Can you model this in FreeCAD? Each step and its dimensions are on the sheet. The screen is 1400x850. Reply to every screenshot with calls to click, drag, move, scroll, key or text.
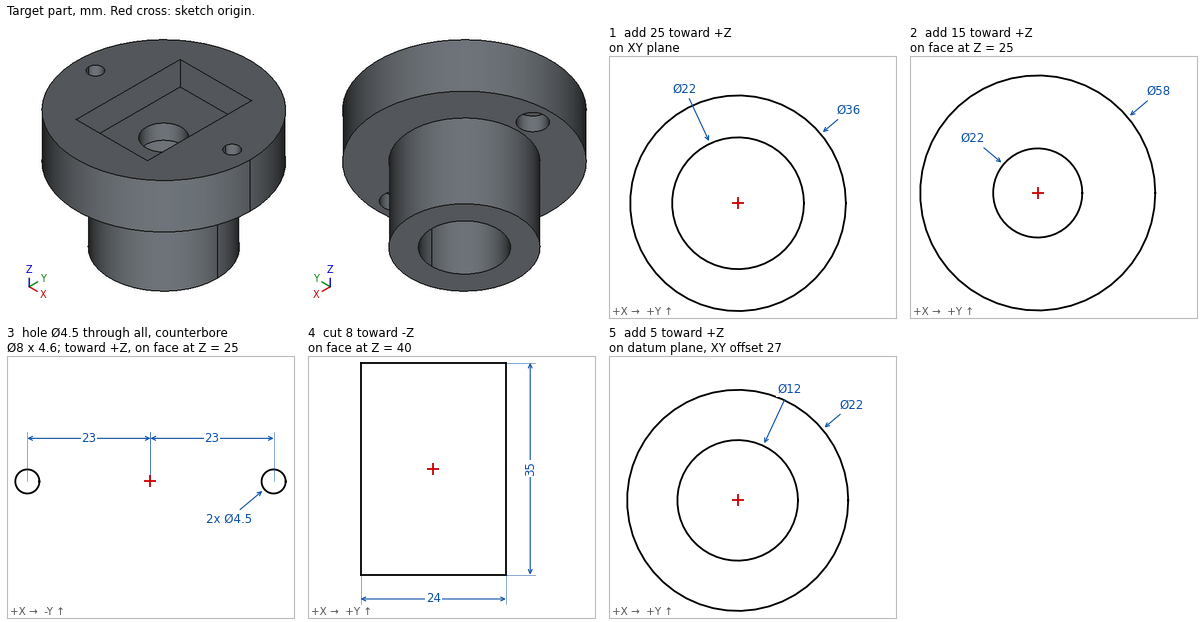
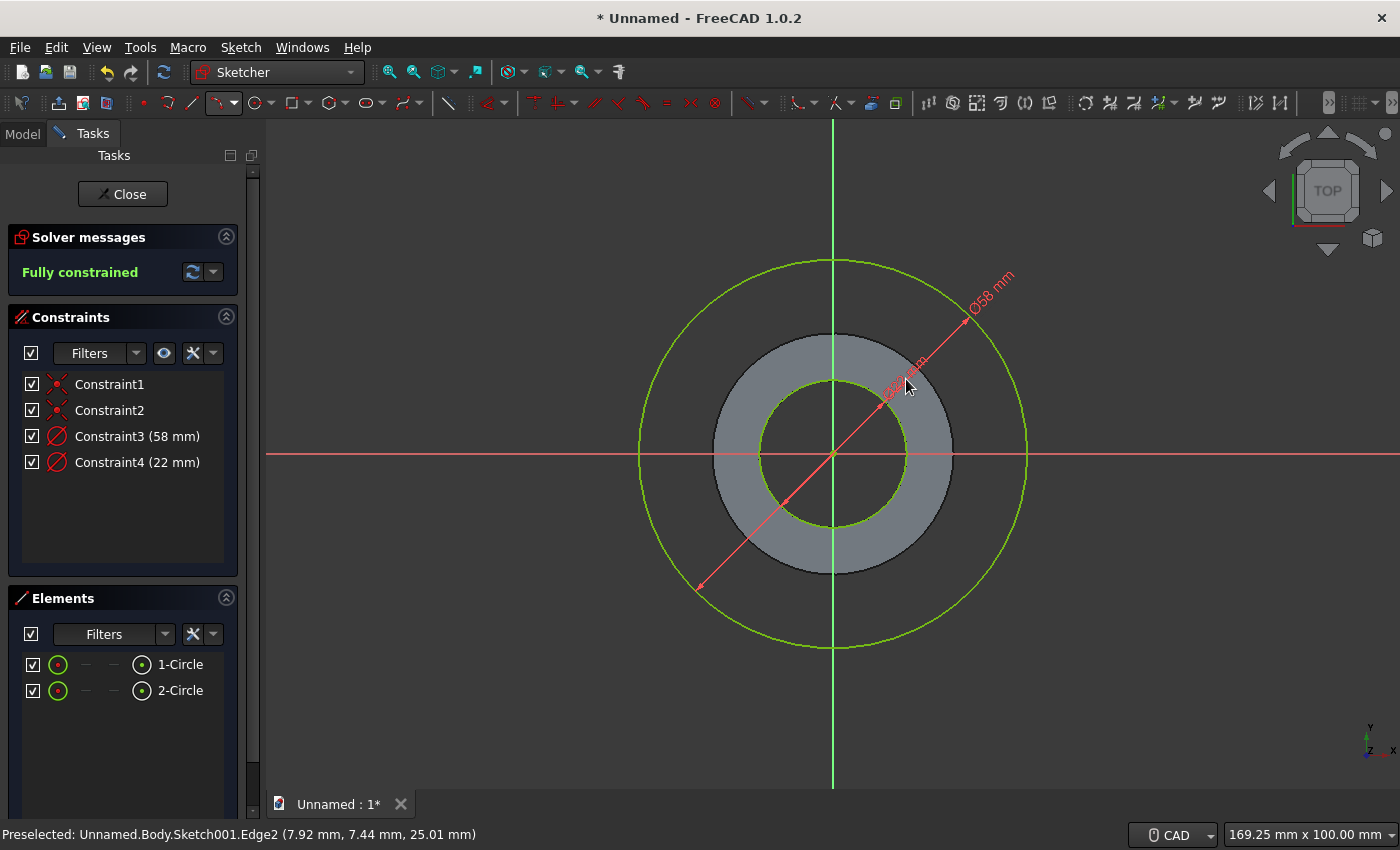
click(123, 194)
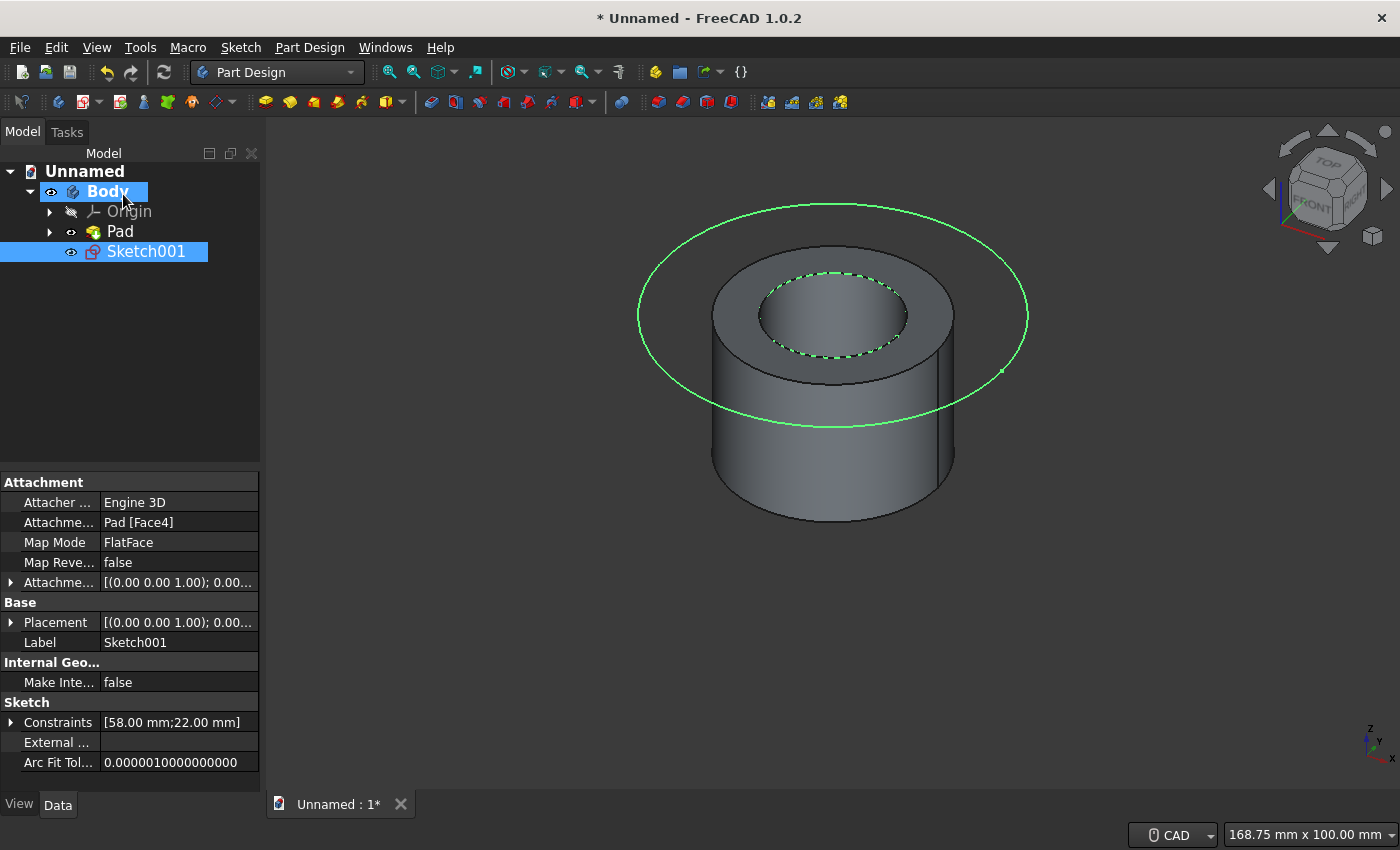
click(266, 102)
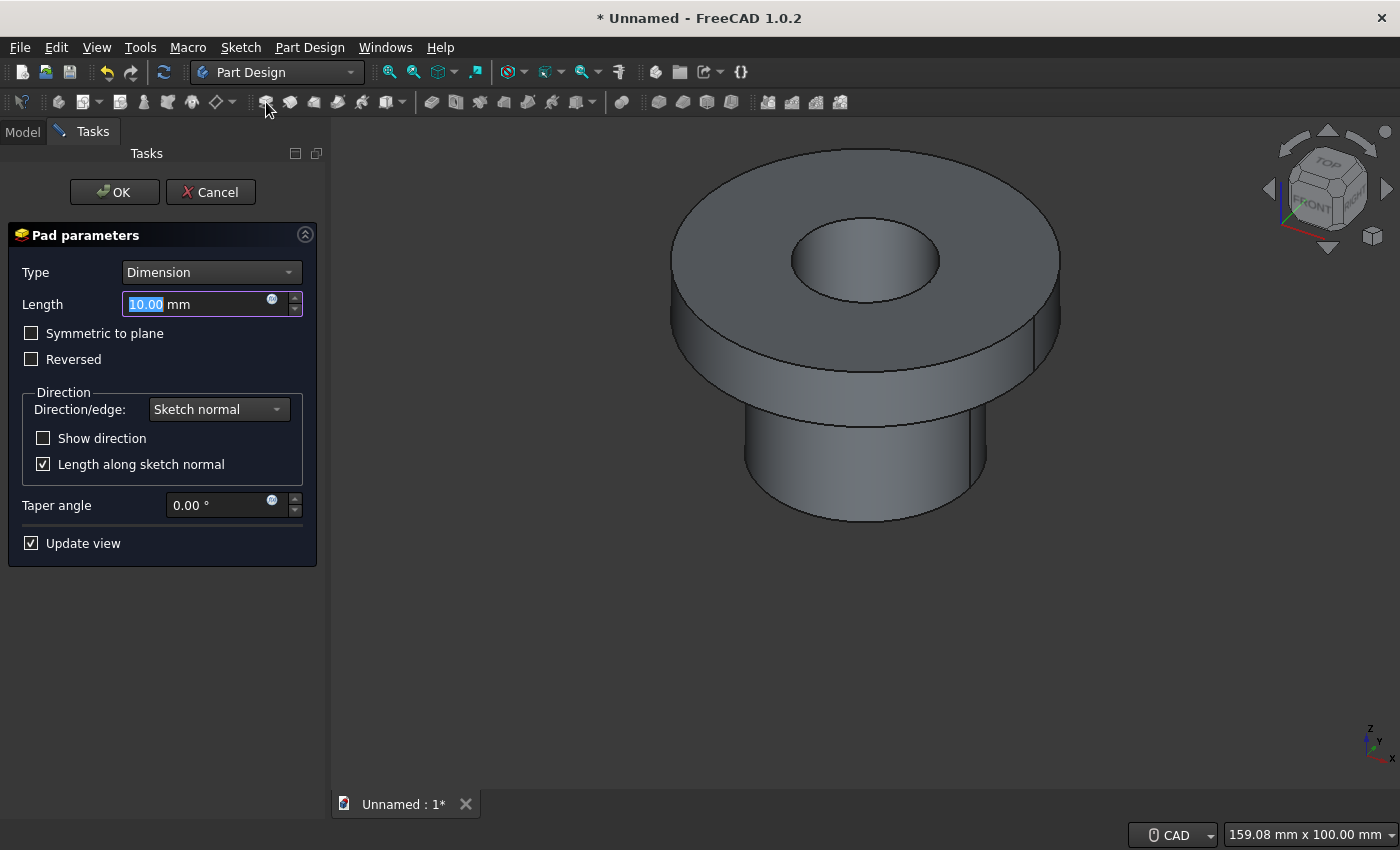
text(15)
key(Tab)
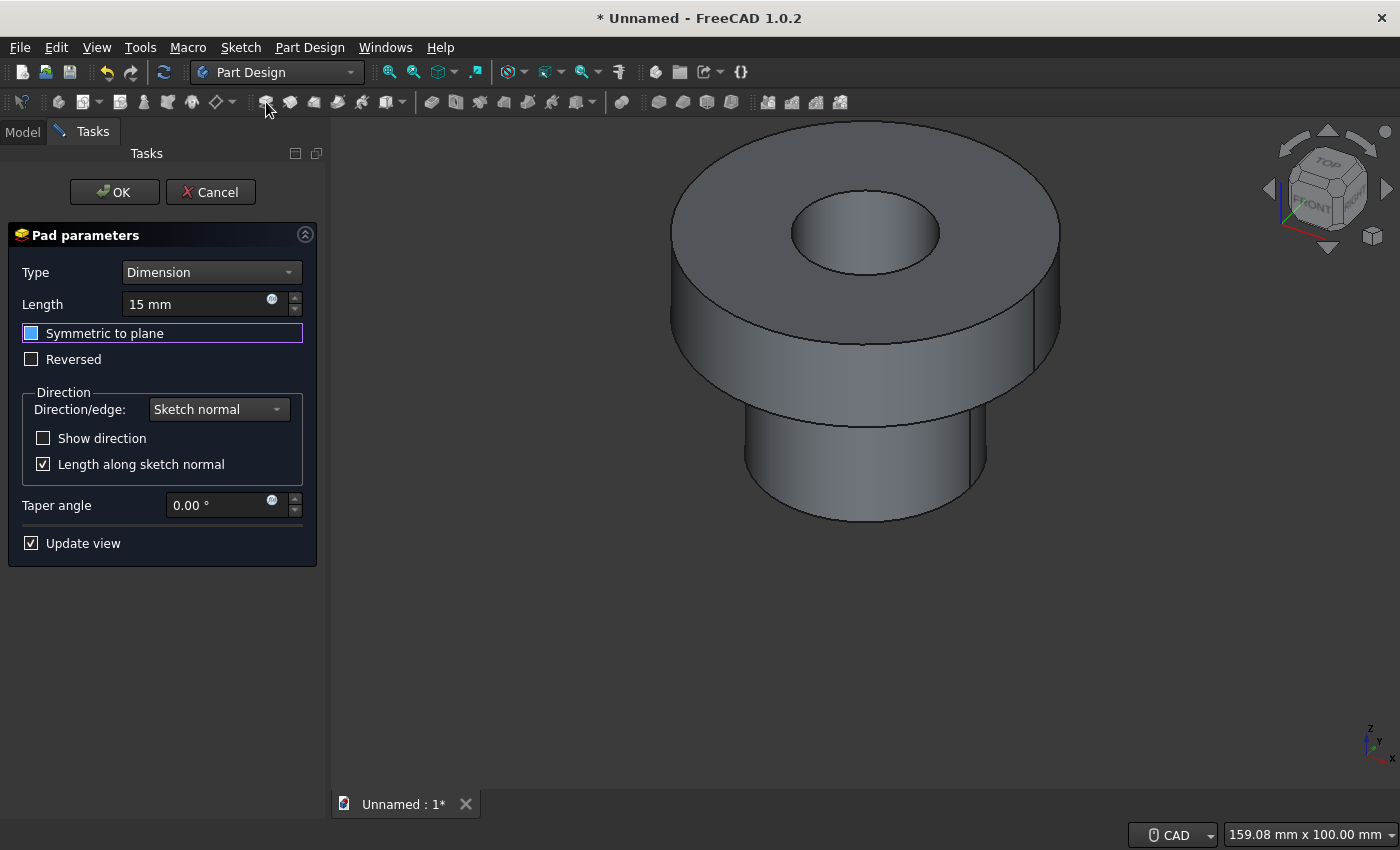
click(115, 192)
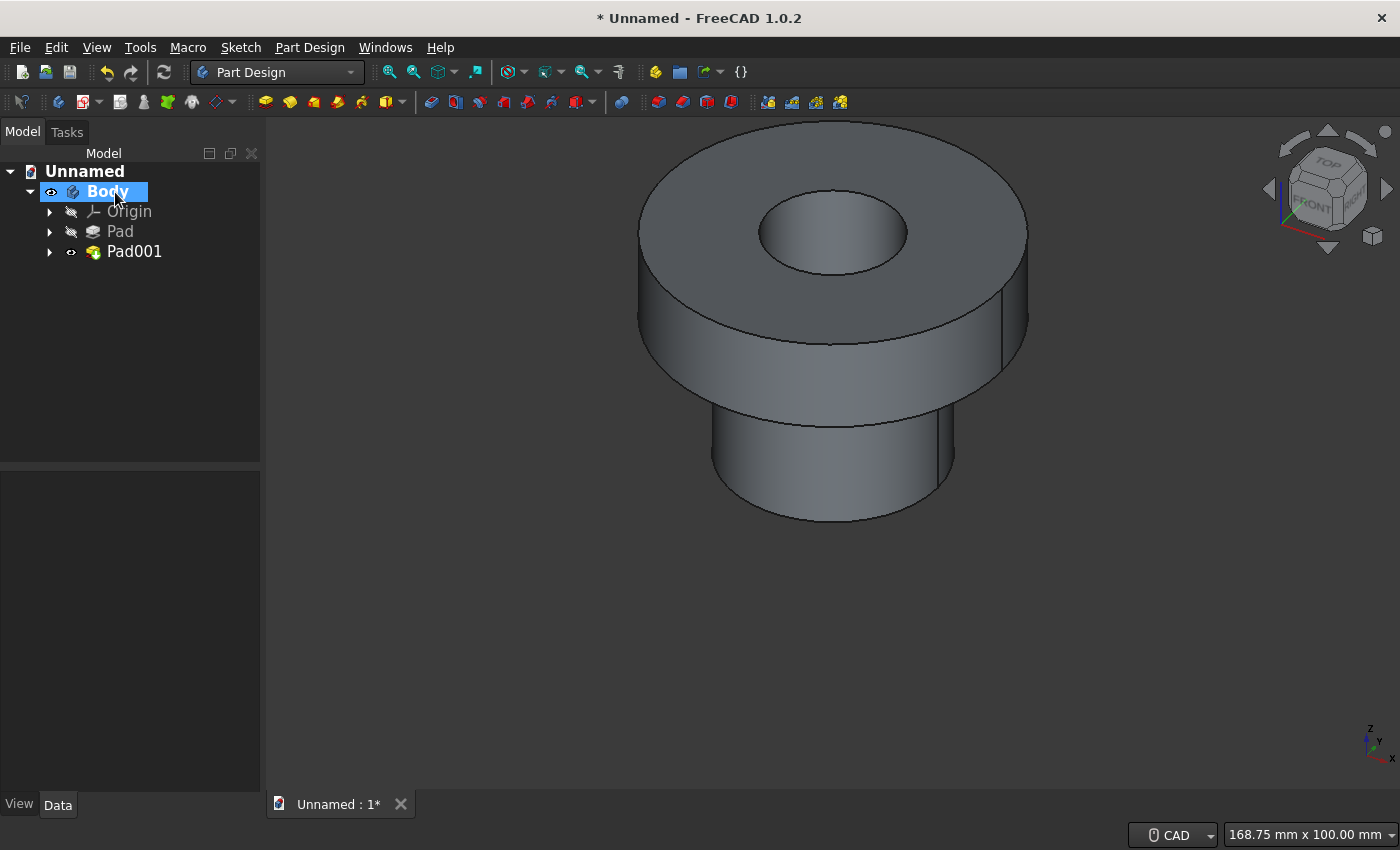
key(v)
key(f)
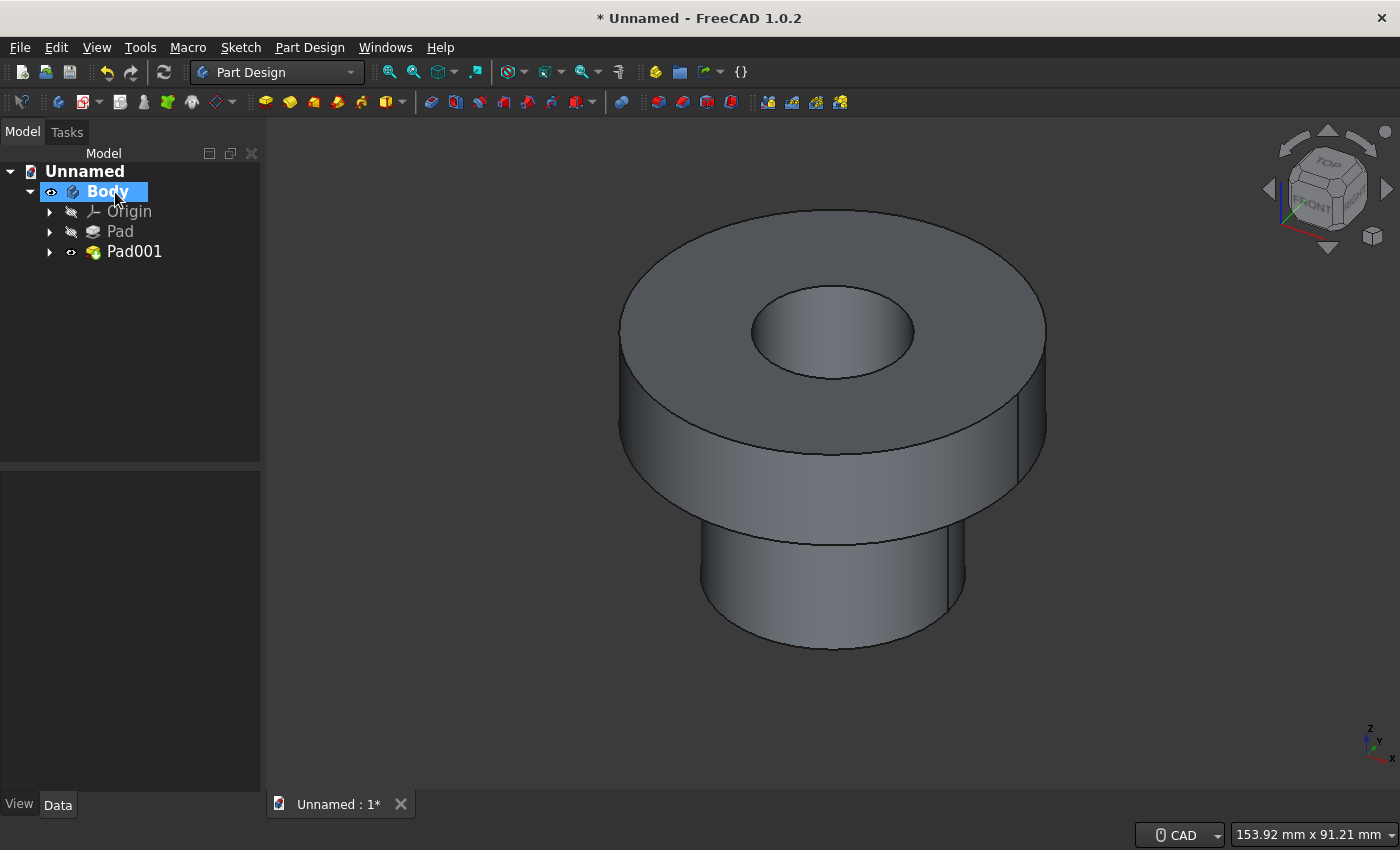
key(5)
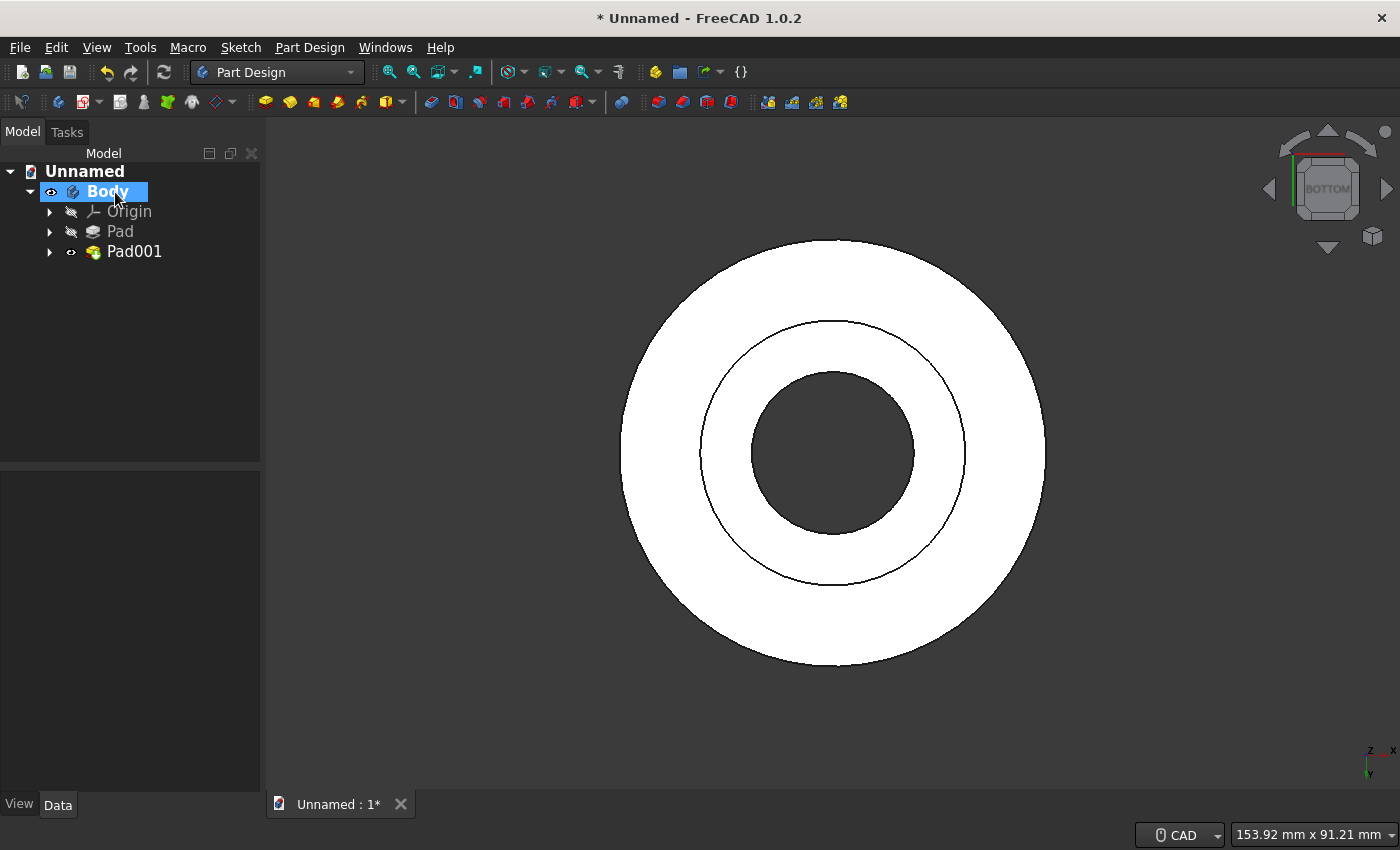
click(955, 330)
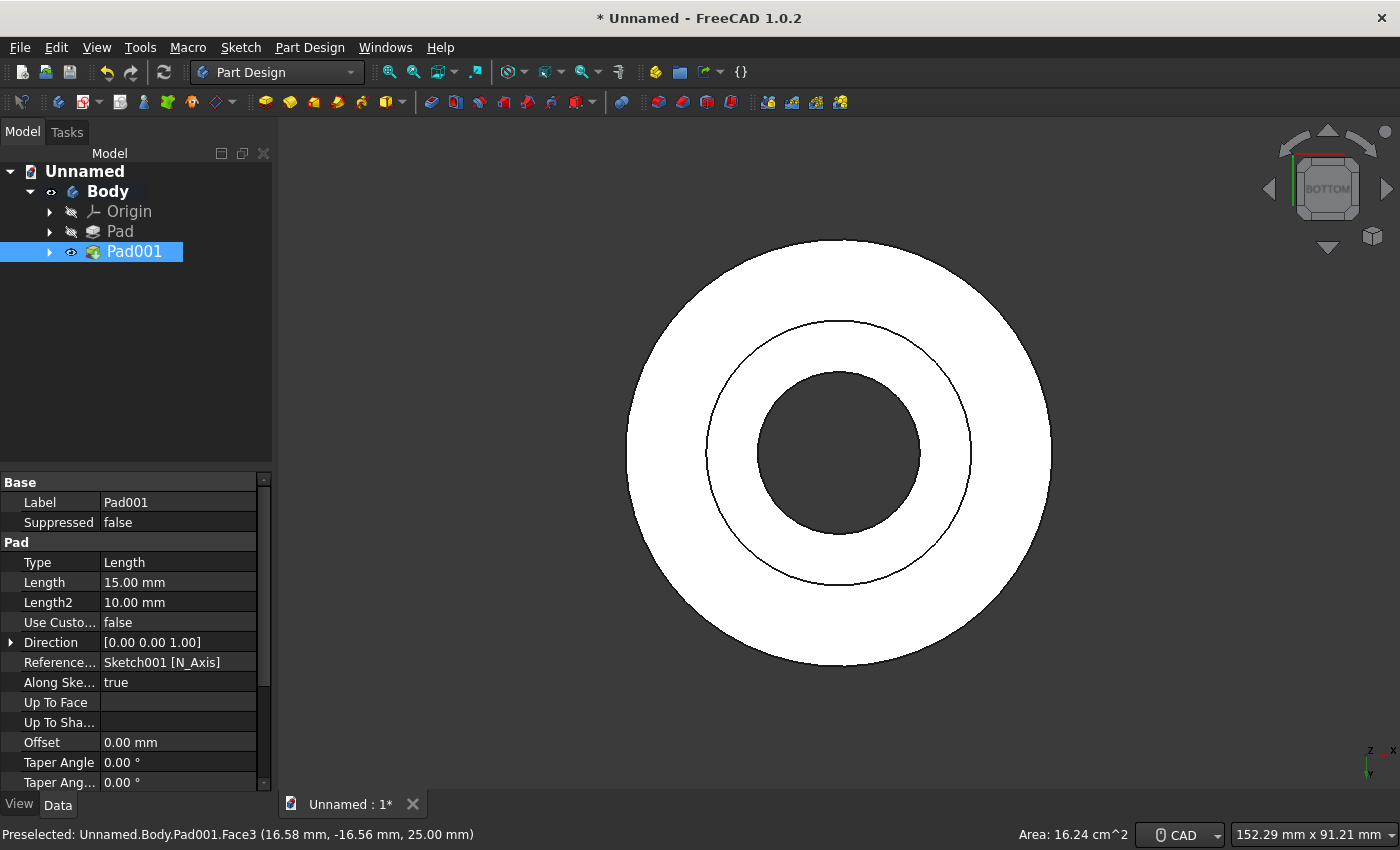
click(84, 102)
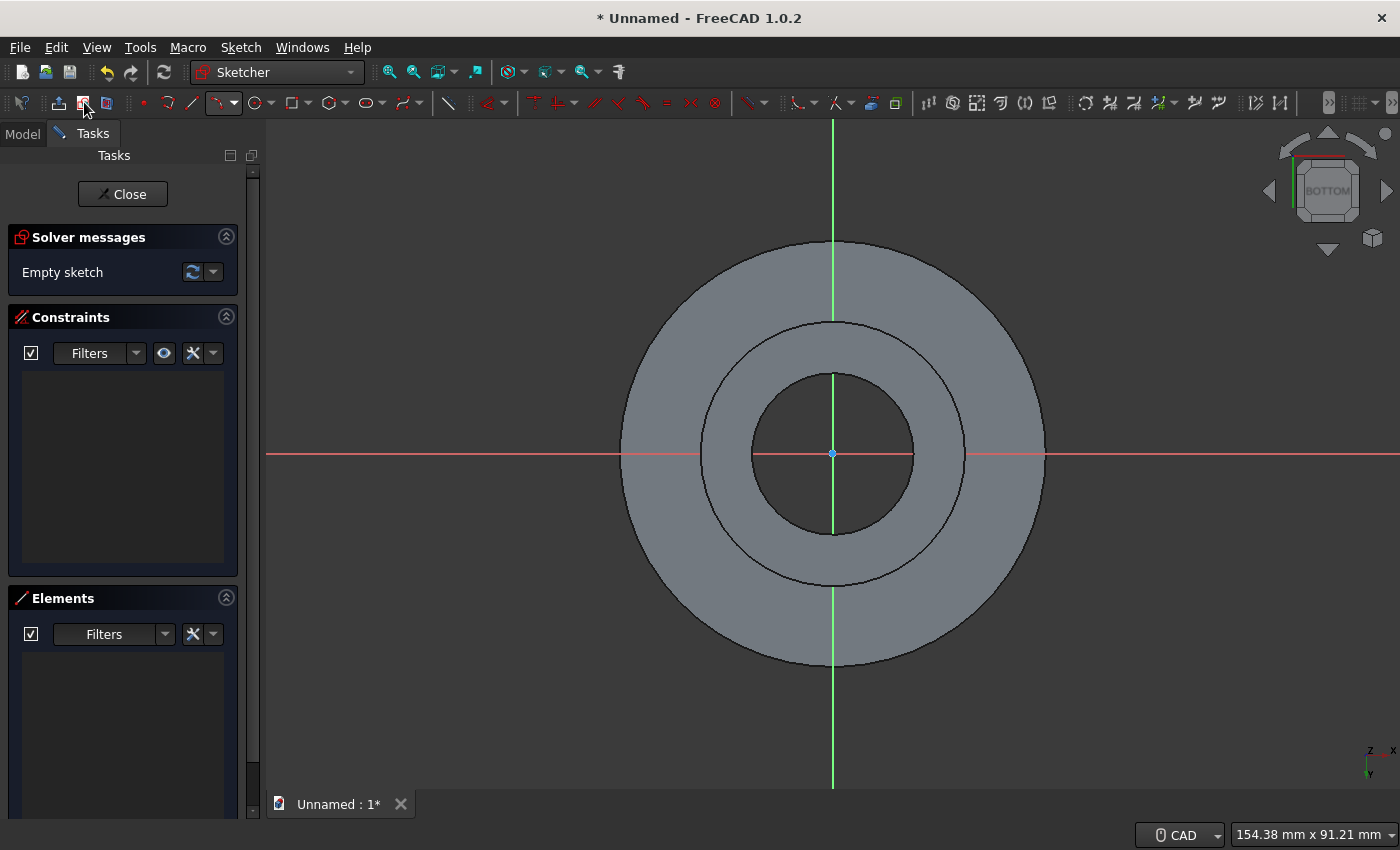
key(q)
key(s)